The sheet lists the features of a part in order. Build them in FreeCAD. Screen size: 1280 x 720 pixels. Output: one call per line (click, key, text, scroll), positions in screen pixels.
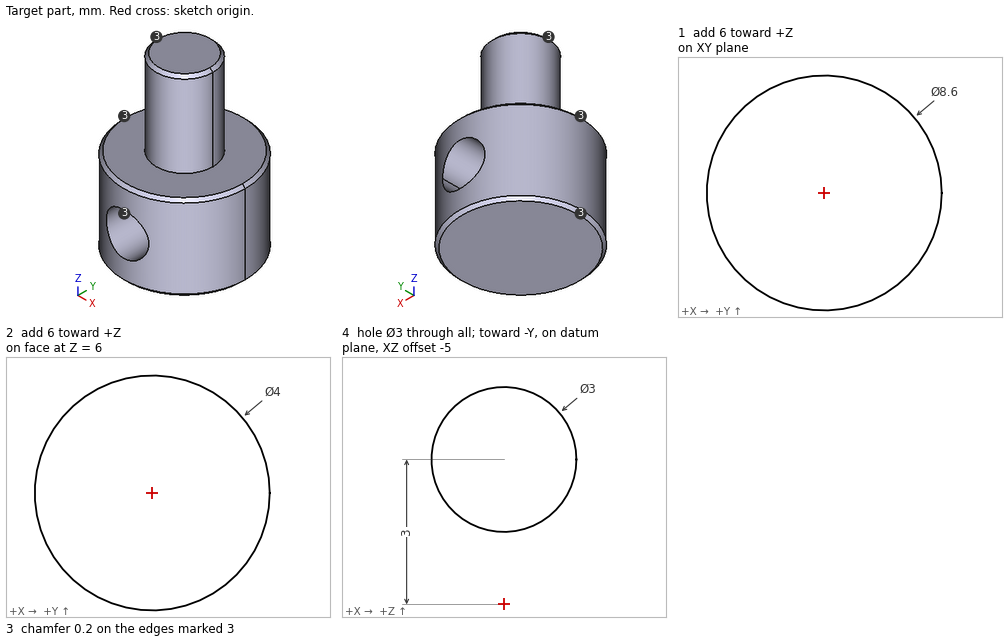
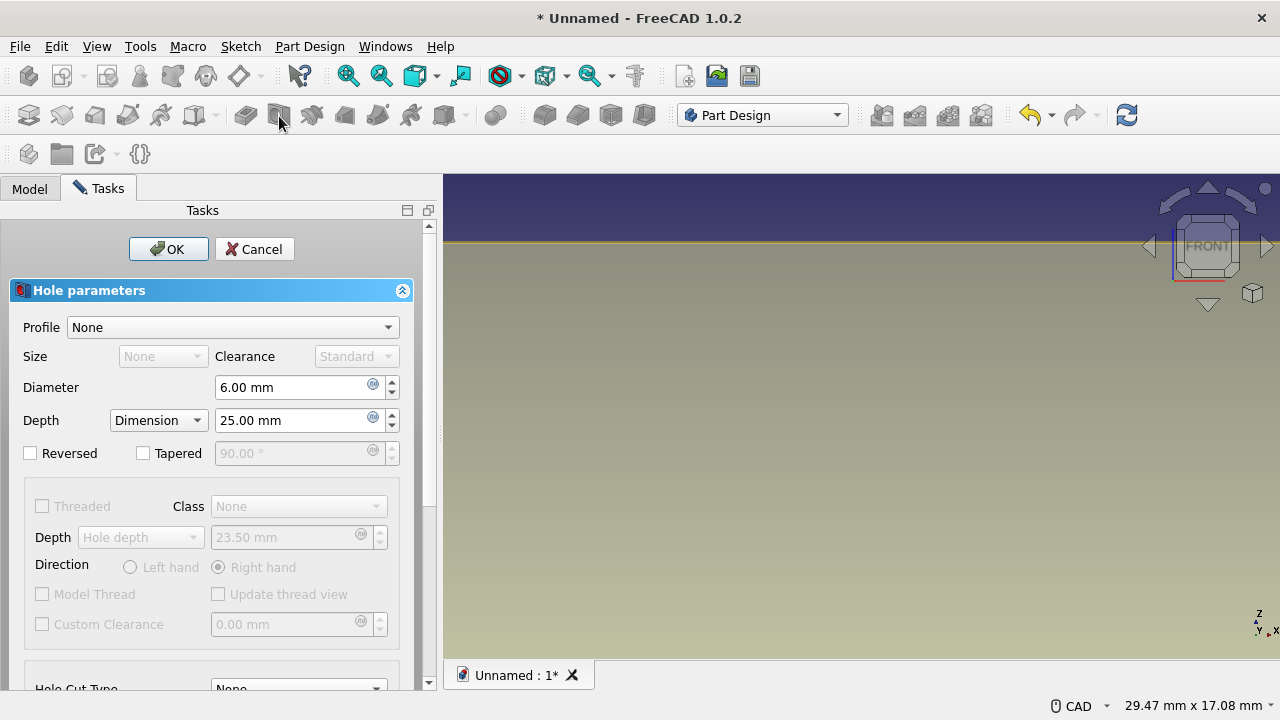
triple_click(300, 388)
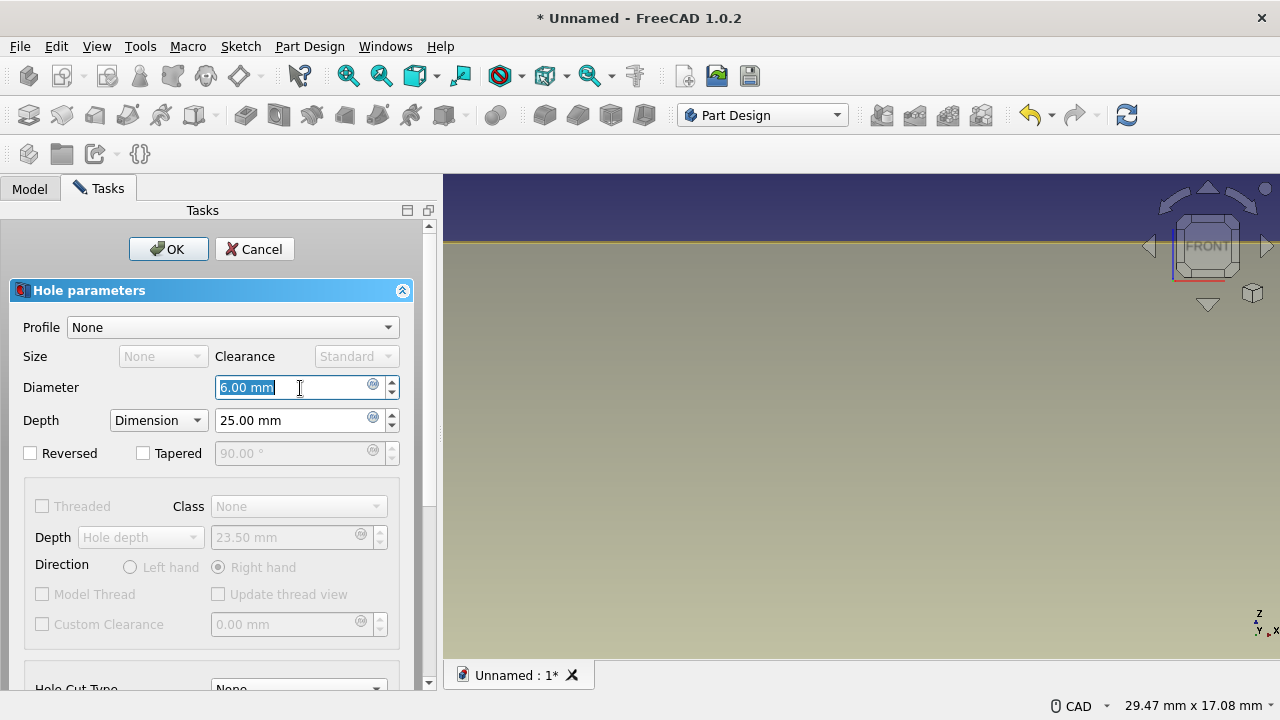
text(3)
key(Tab)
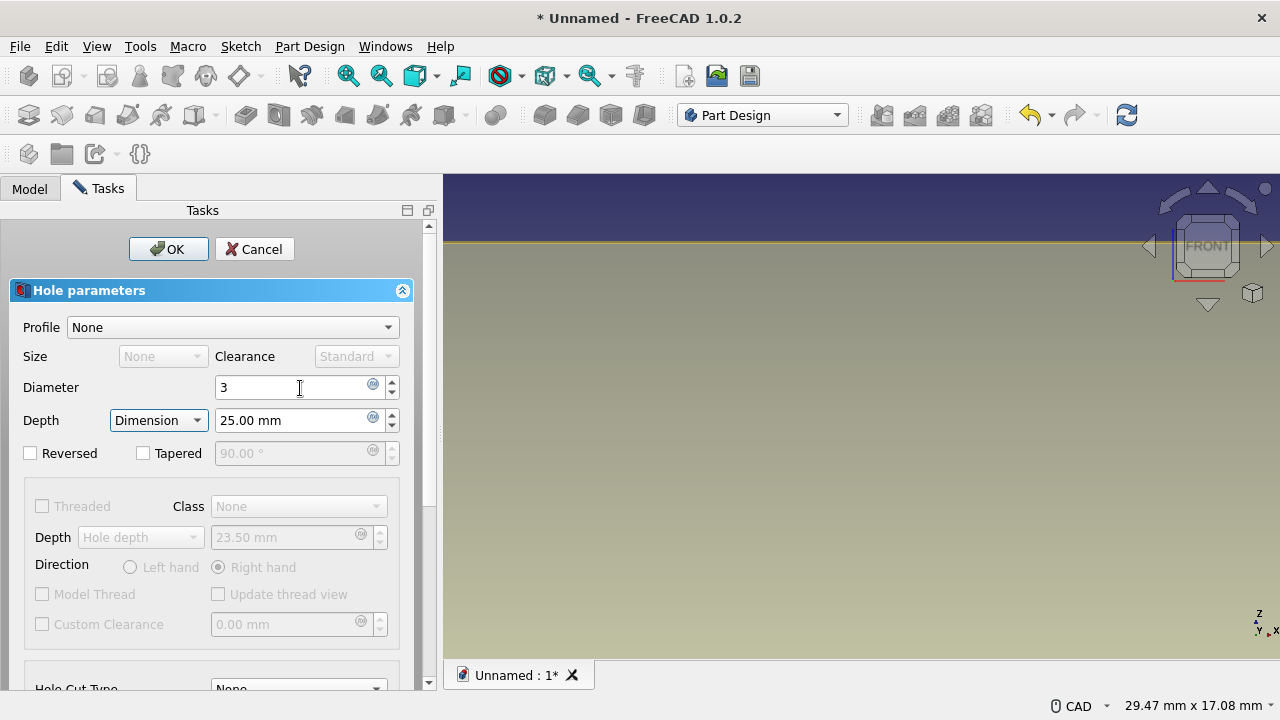
click(160, 420)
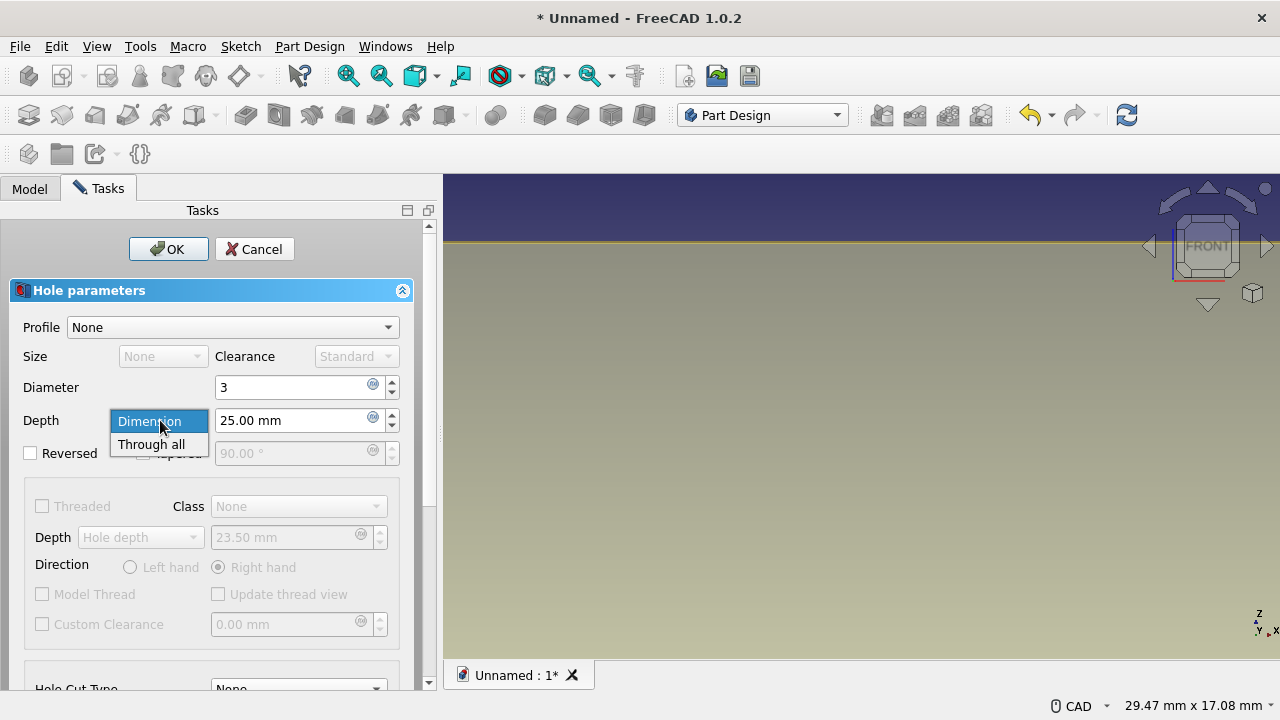
click(158, 444)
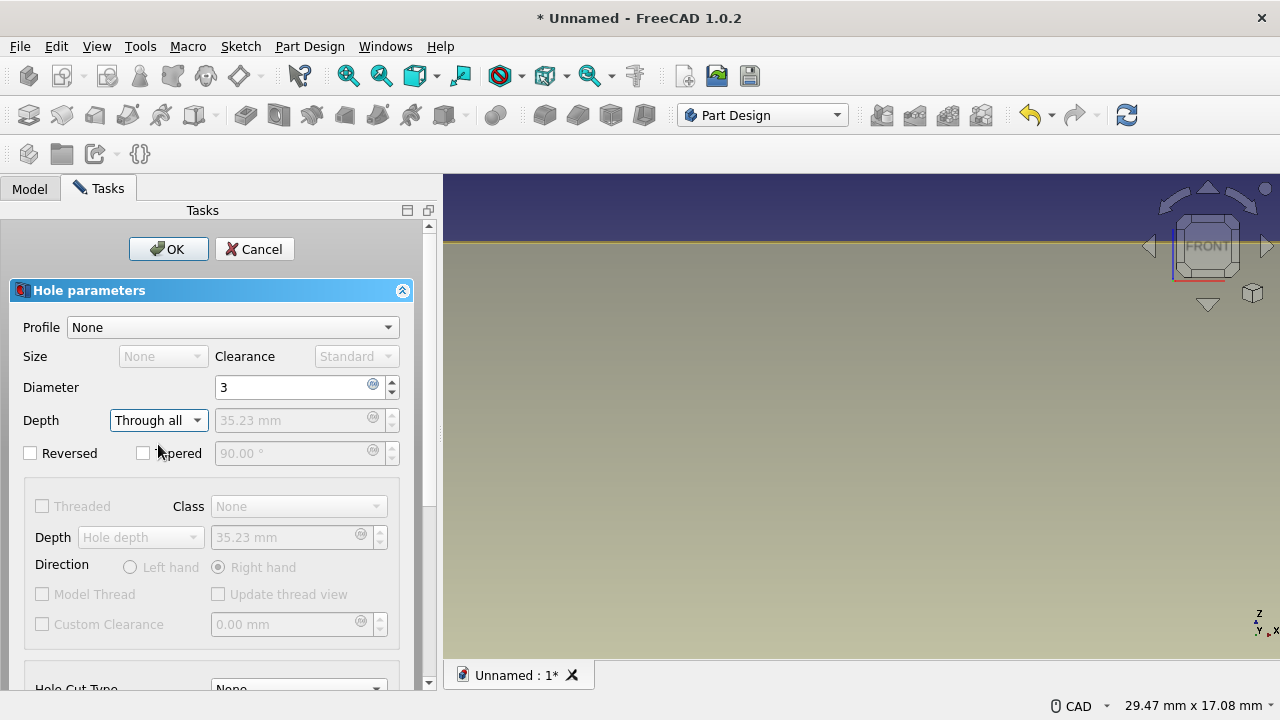
click(31, 453)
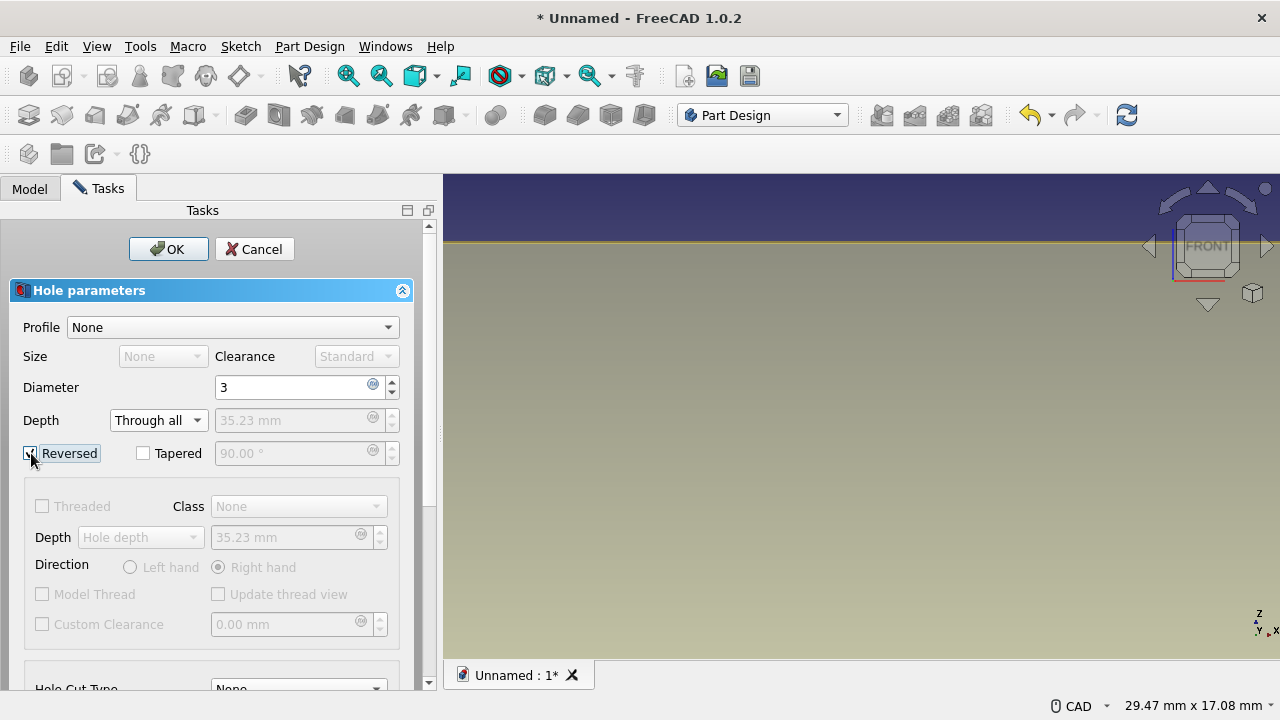
click(169, 249)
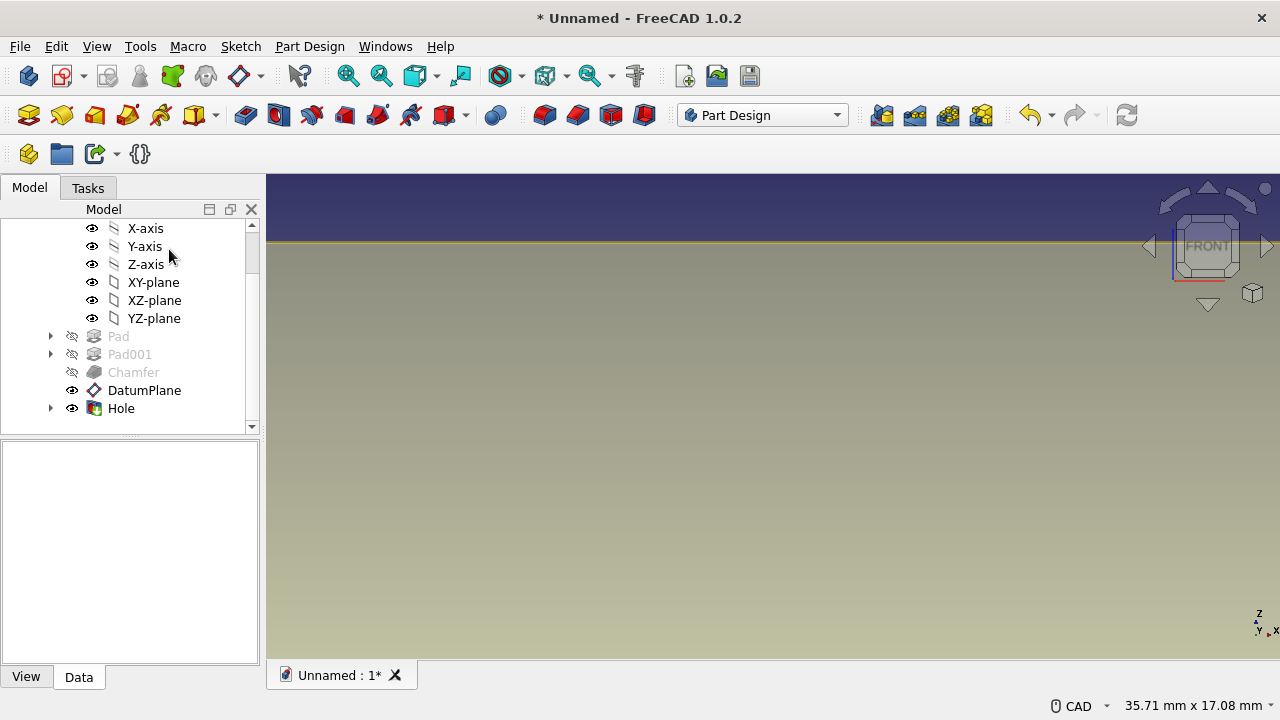
click(117, 390)
key(space)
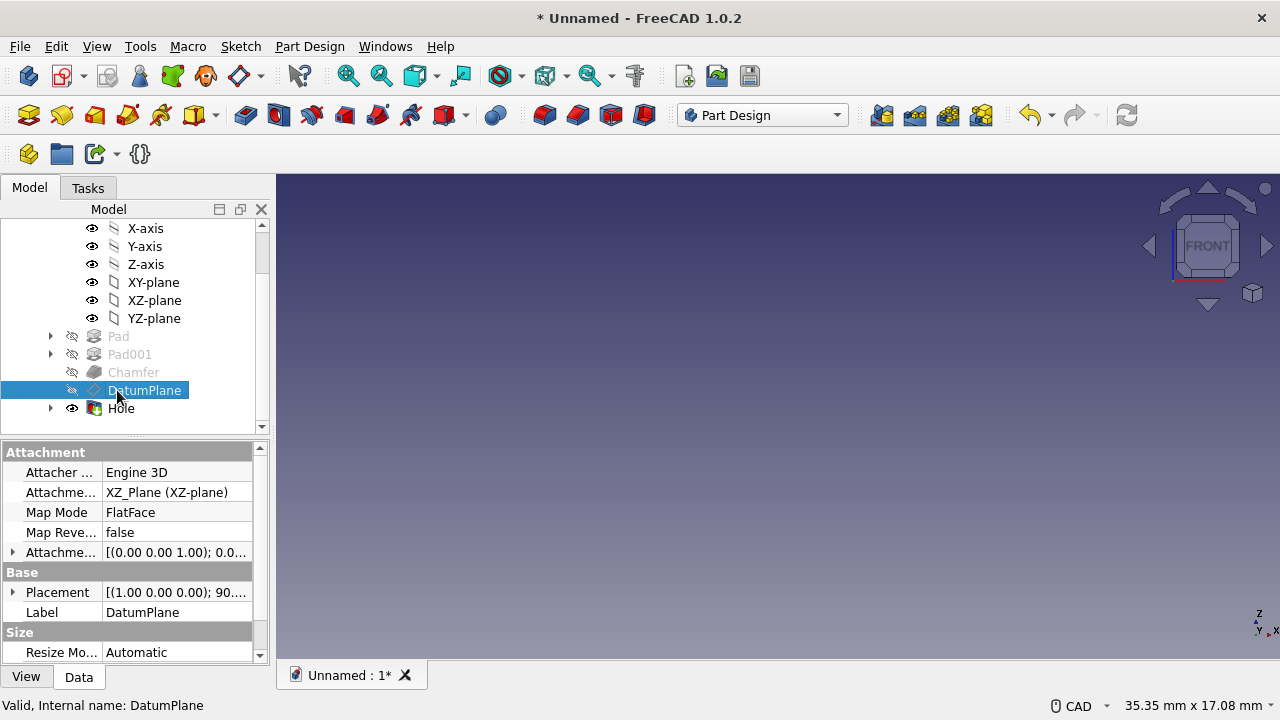
key(0)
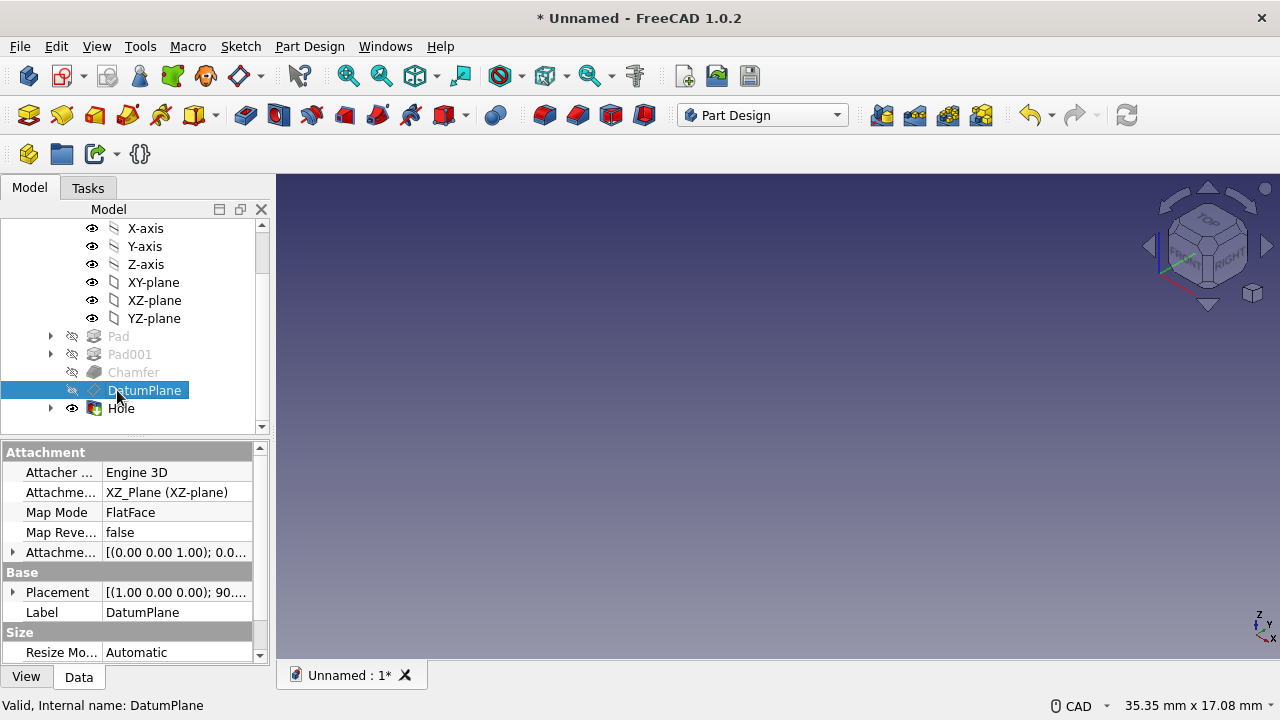
key(v)
key(f)